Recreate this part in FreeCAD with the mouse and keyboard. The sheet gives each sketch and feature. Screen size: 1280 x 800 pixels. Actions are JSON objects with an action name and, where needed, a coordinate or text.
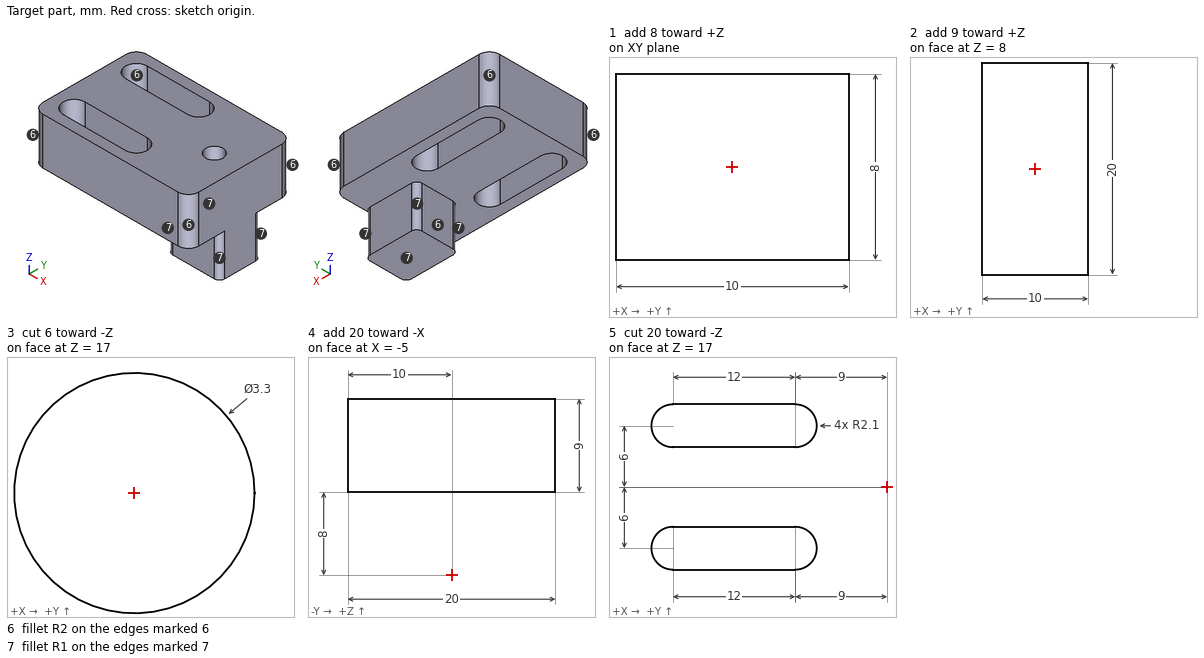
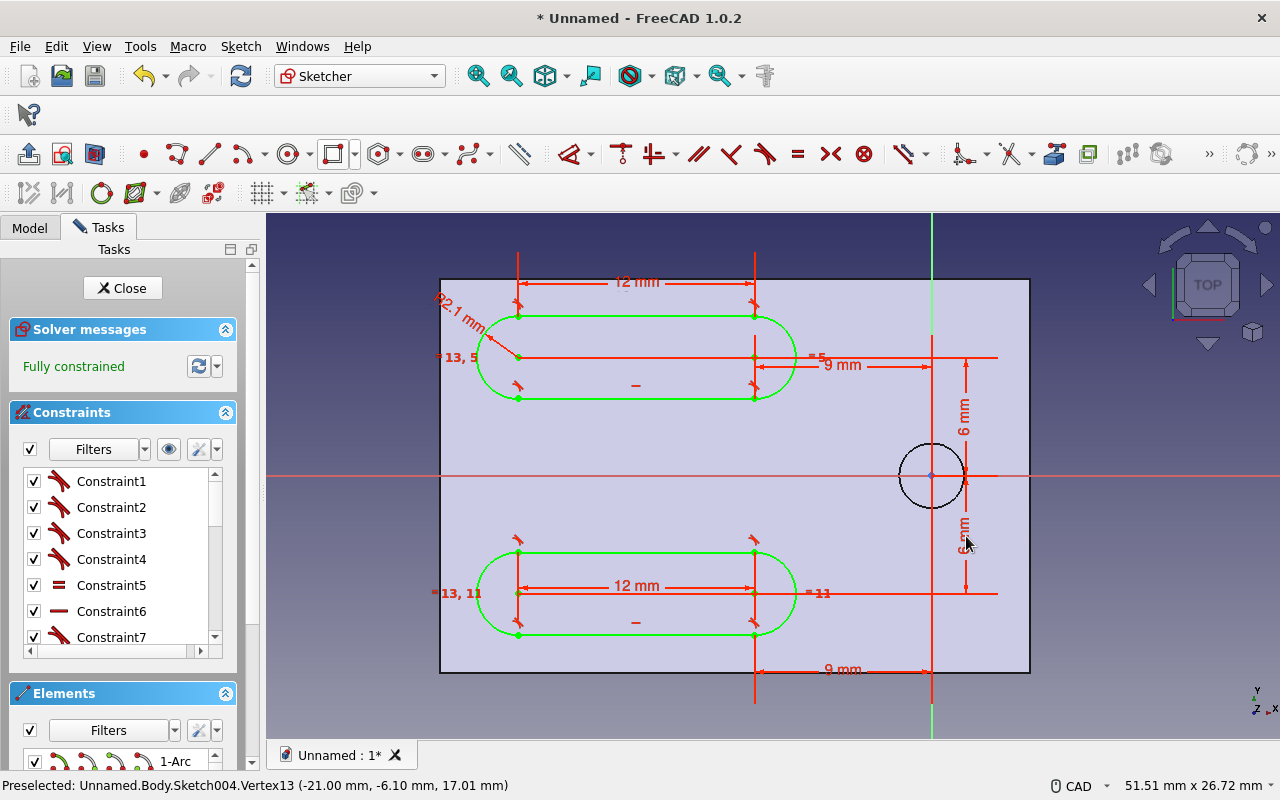
{"action": "left_click", "coordinate": [123, 288]}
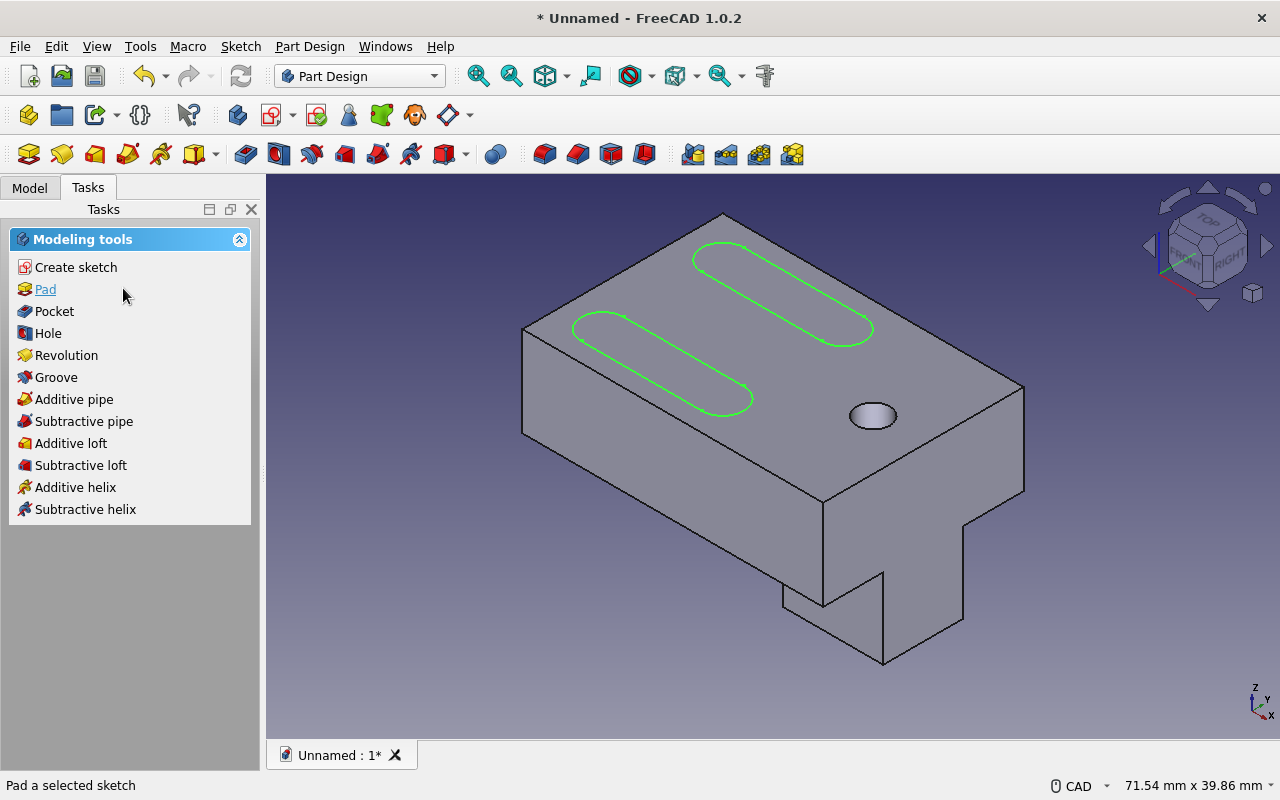
{"action": "left_click", "coordinate": [246, 154]}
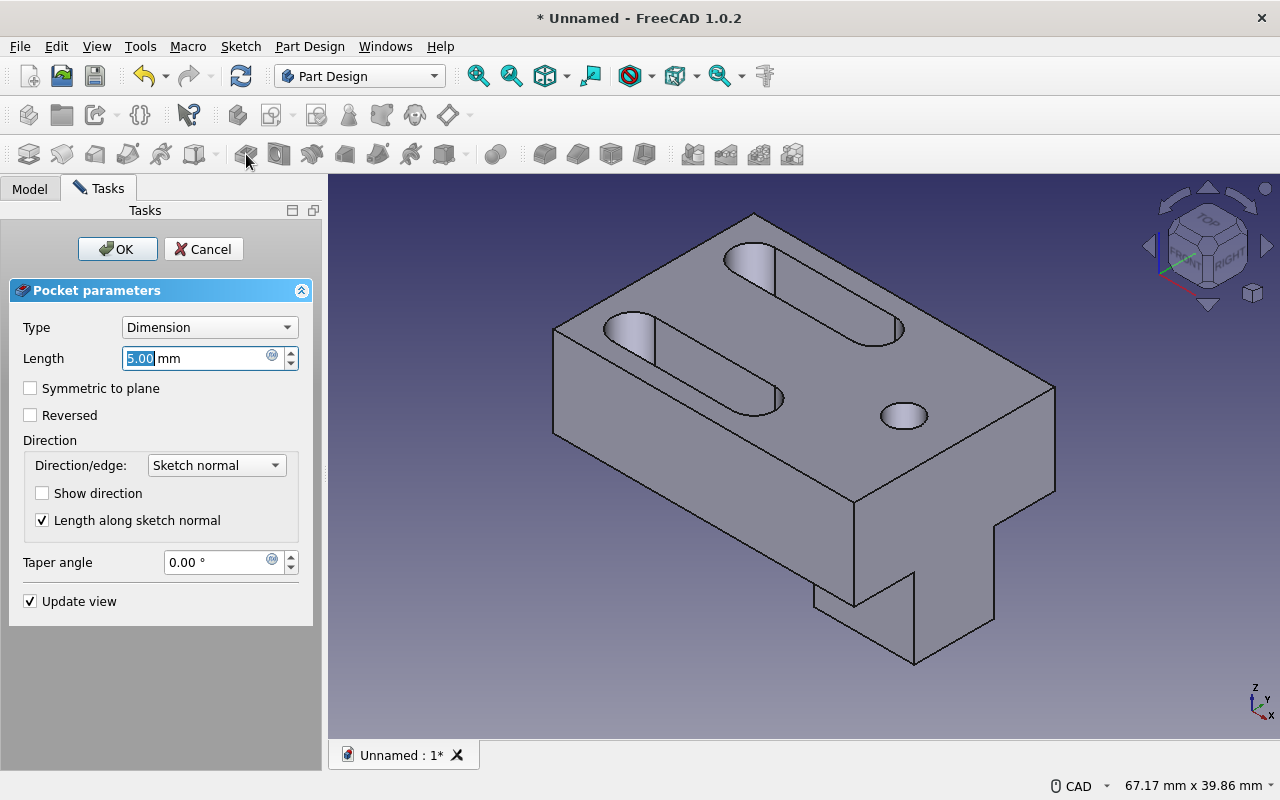
{"action": "type", "text": "20"}
{"action": "key", "text": "Tab"}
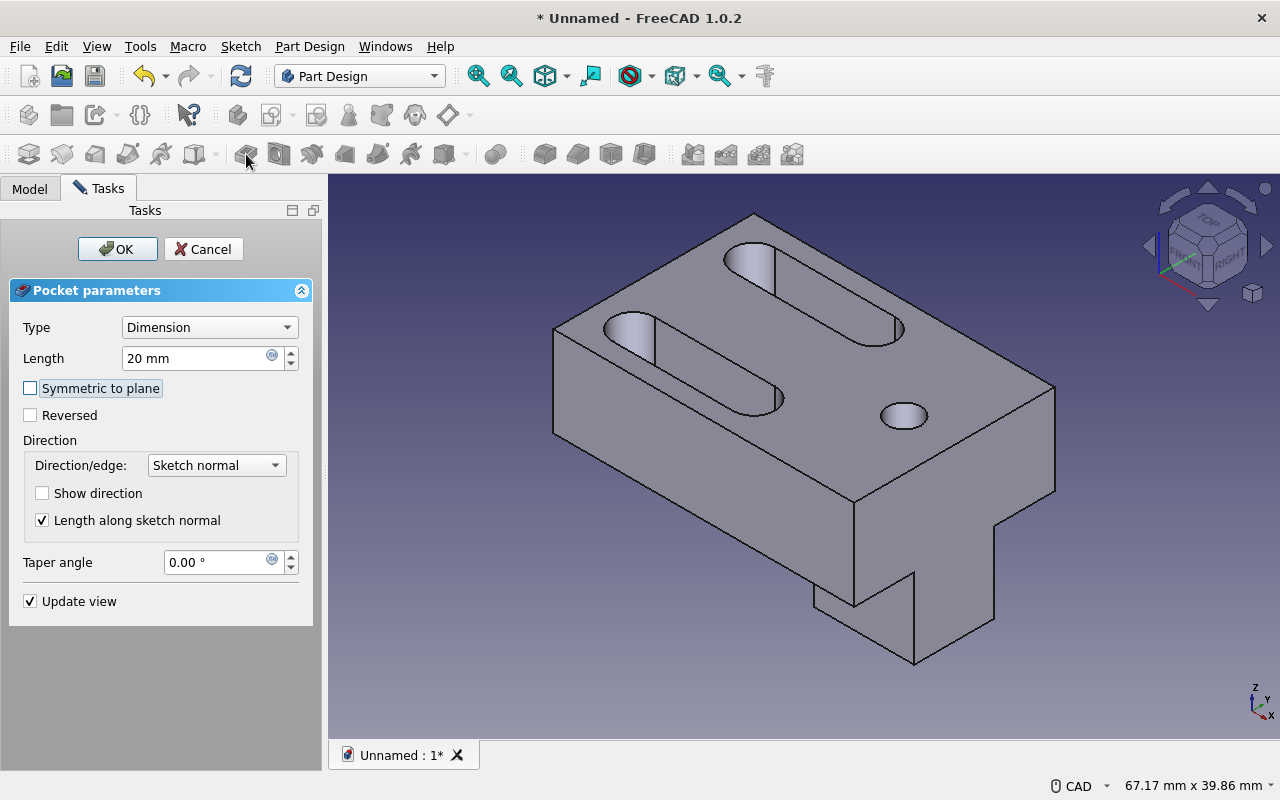
{"action": "left_click", "coordinate": [118, 249]}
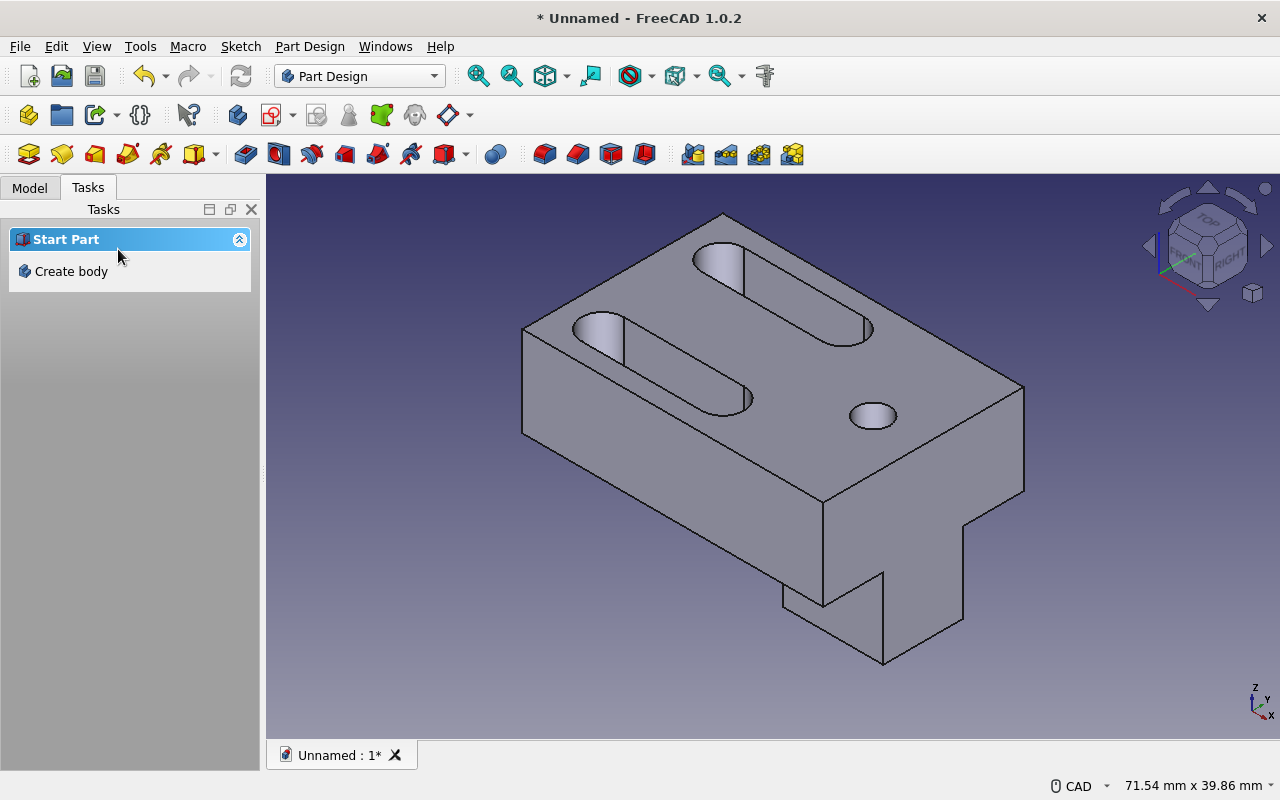
{"action": "left_click", "coordinate": [823, 554]}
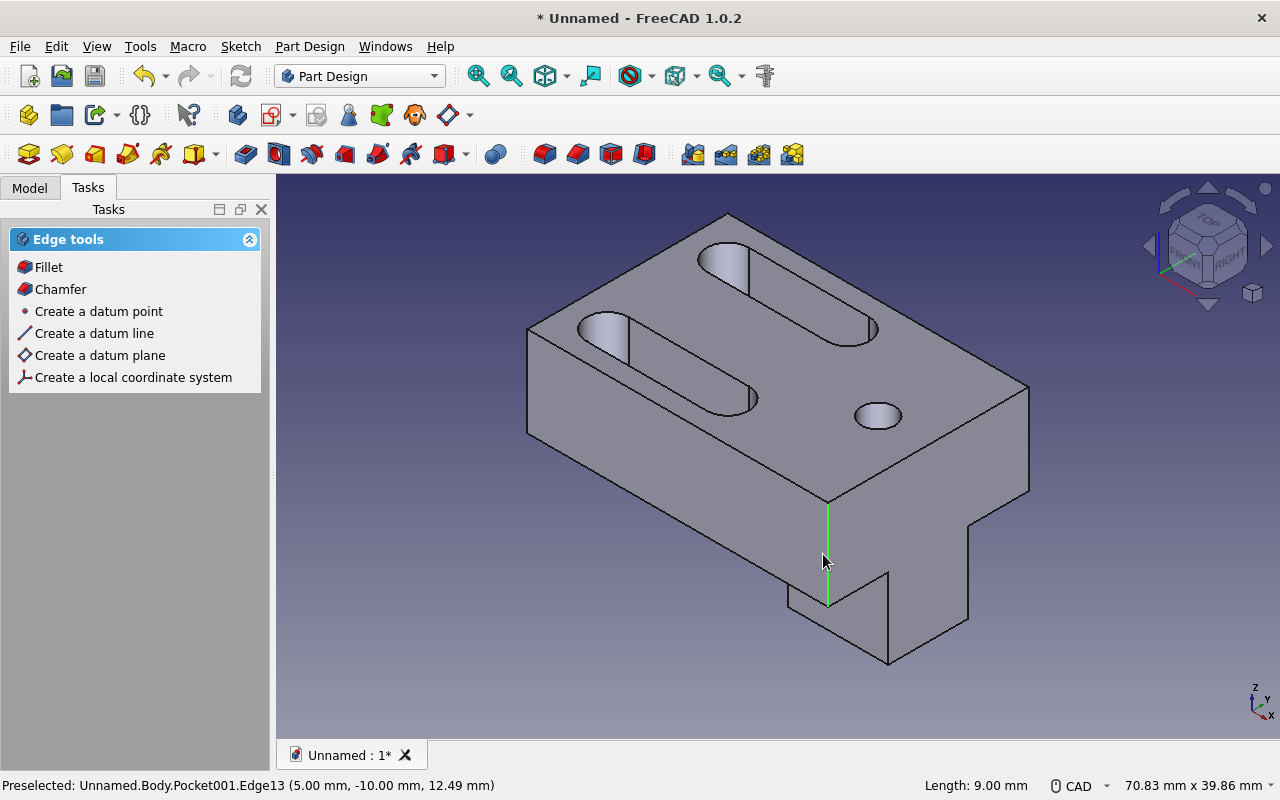
{"action": "key", "text": "2"}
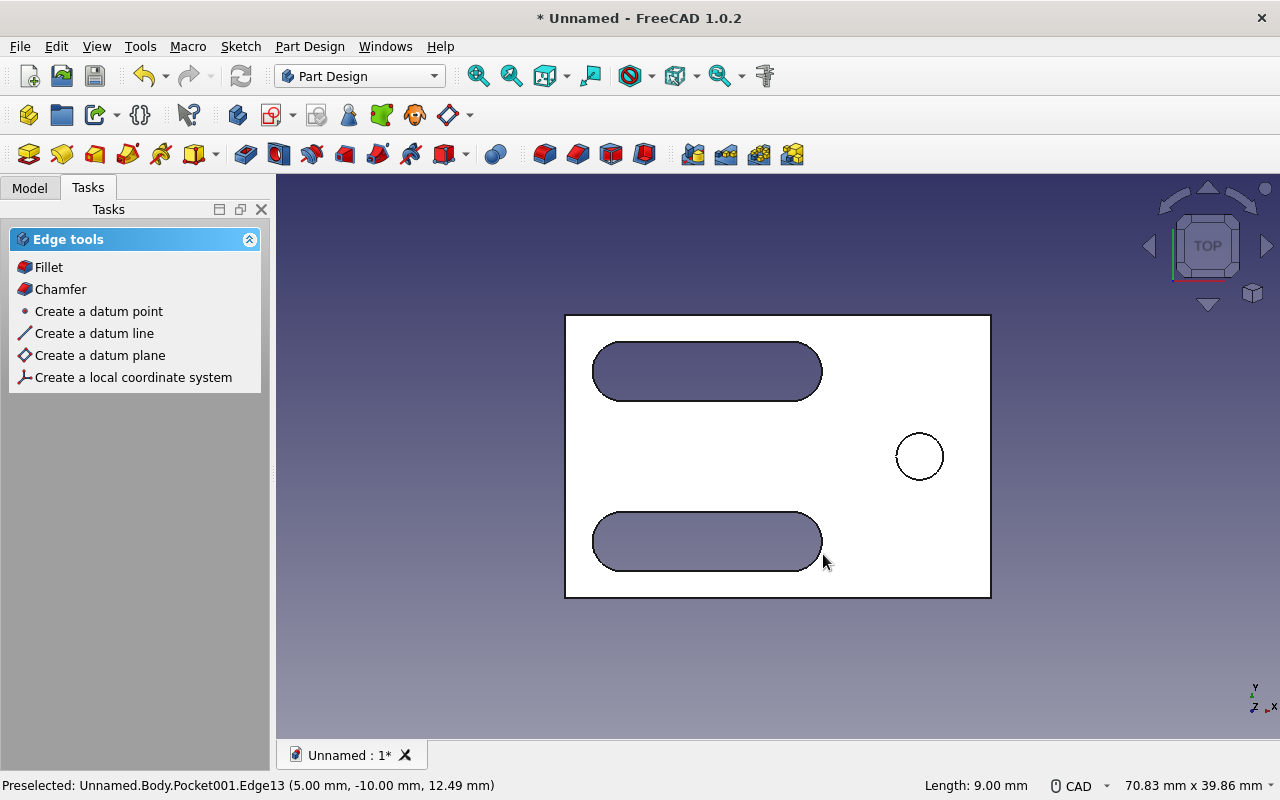
{"action": "key", "text": "0"}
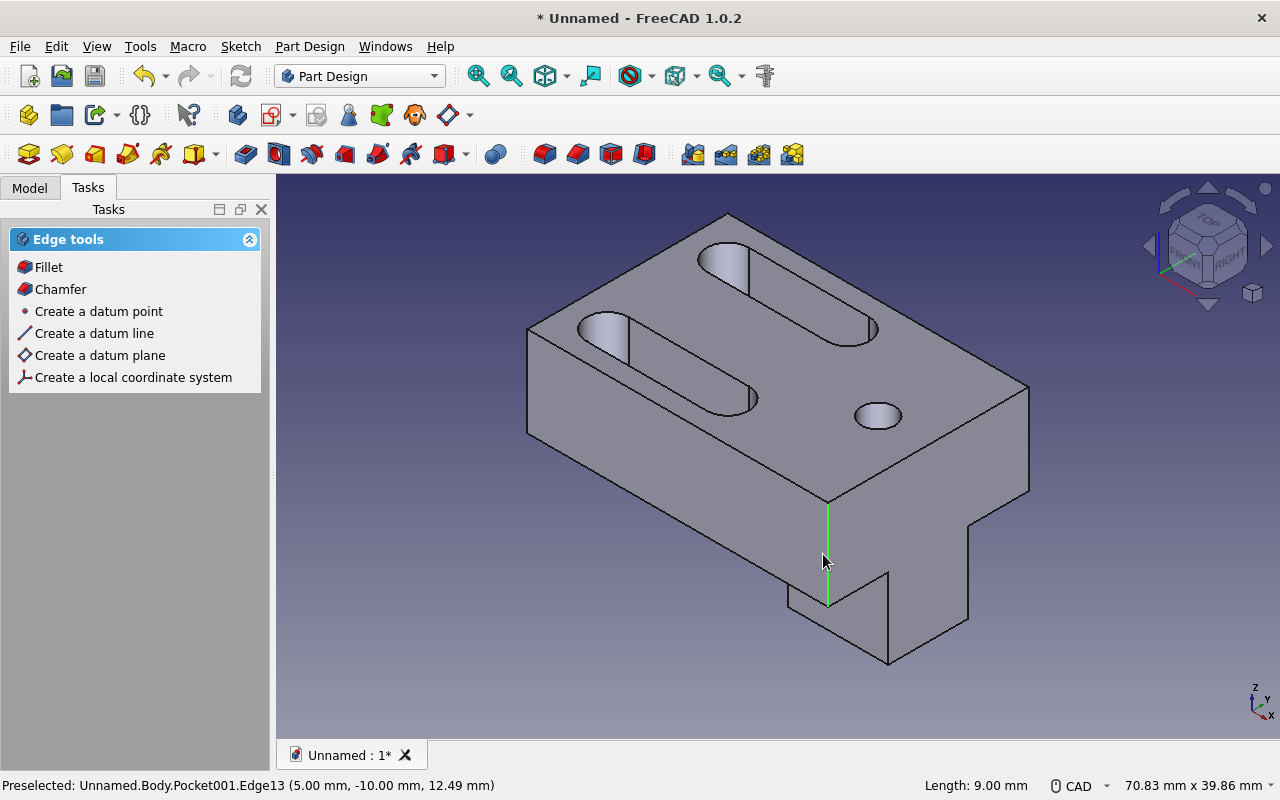
{"action": "key", "text": "1"}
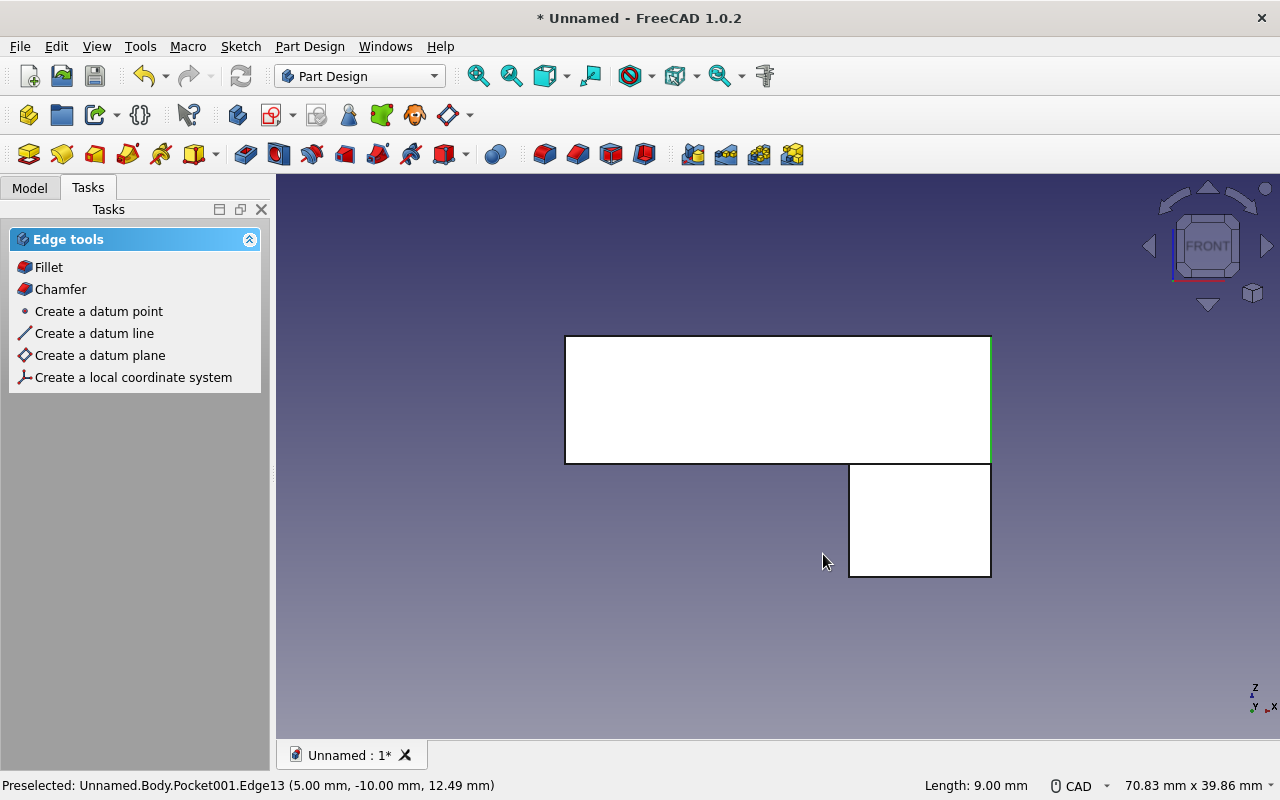
{"action": "key", "text": "v f"}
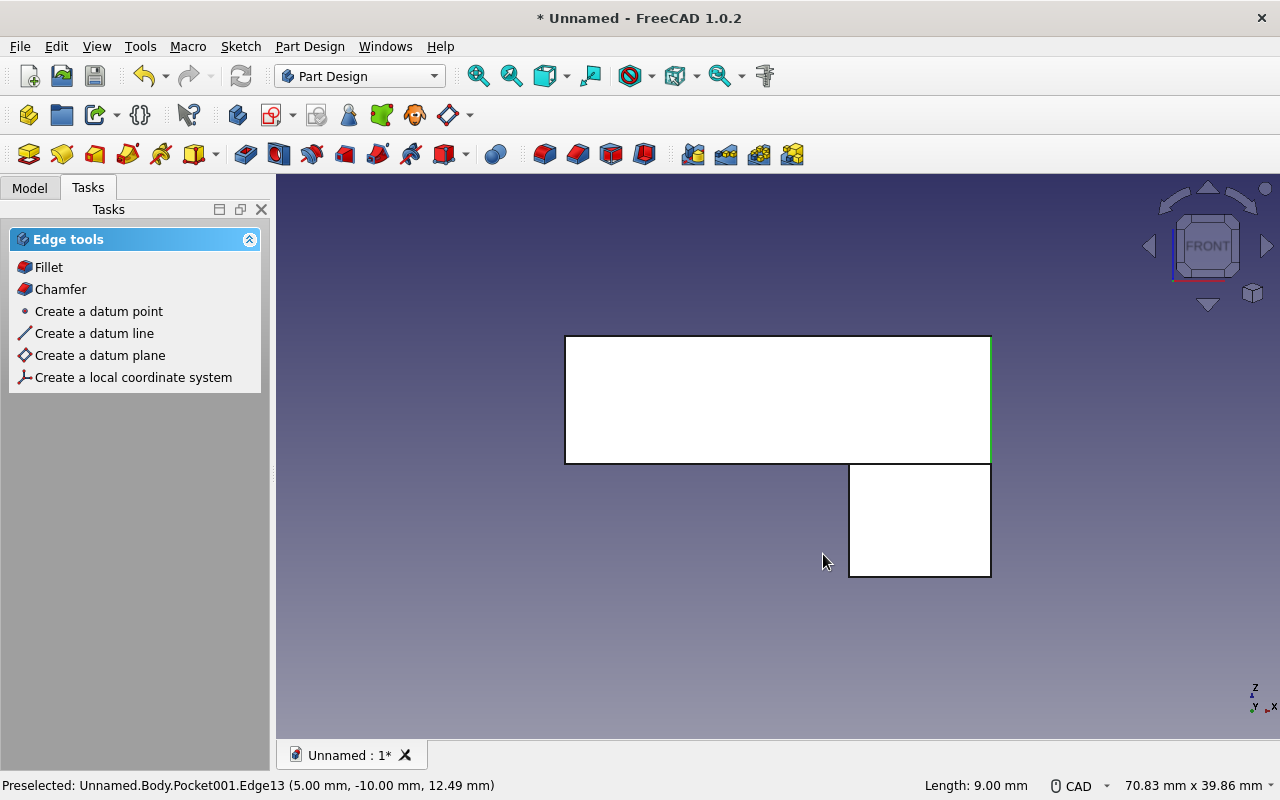
{"action": "left_click", "coordinate": [565, 399], "text": "ctrl"}